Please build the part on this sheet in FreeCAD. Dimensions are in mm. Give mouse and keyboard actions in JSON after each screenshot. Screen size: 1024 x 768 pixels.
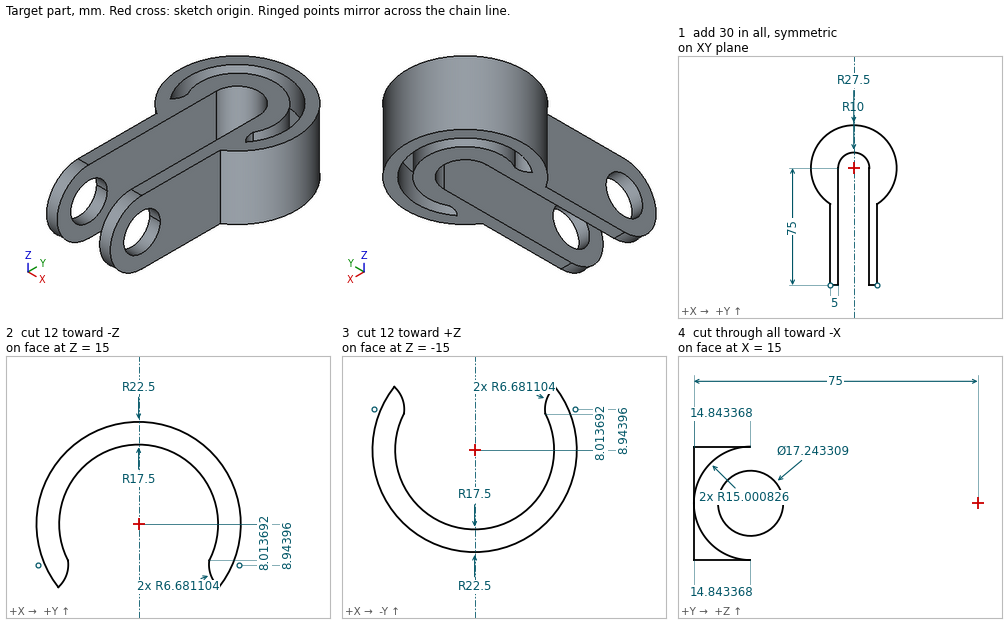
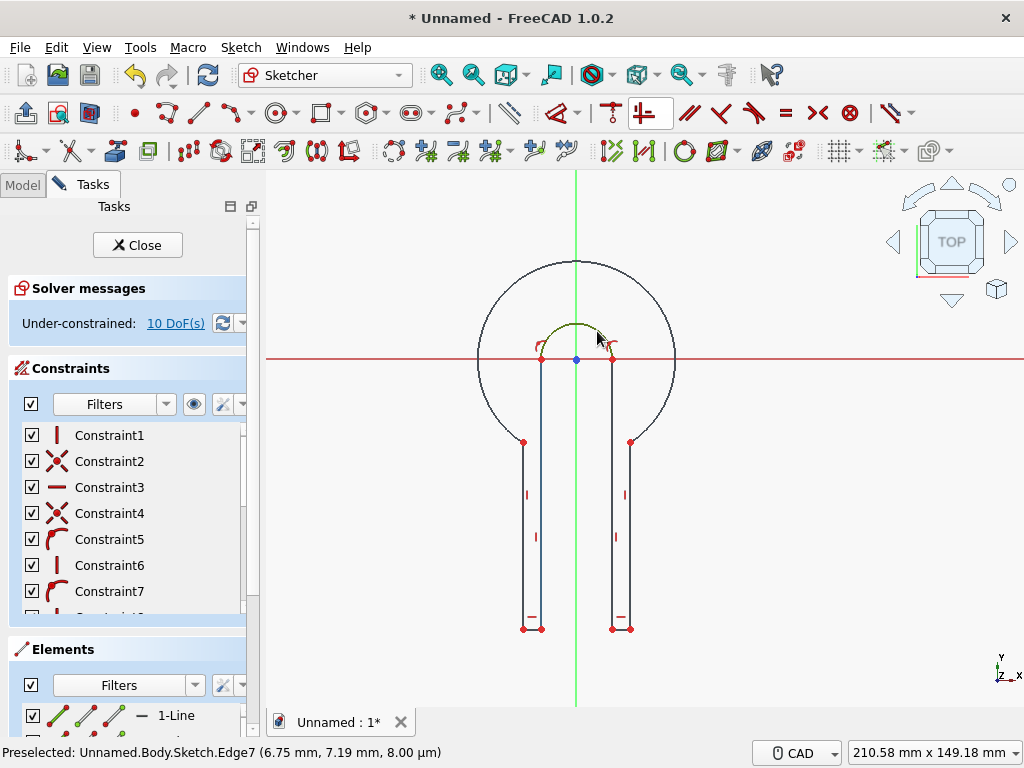
{"action": "key", "text": "t"}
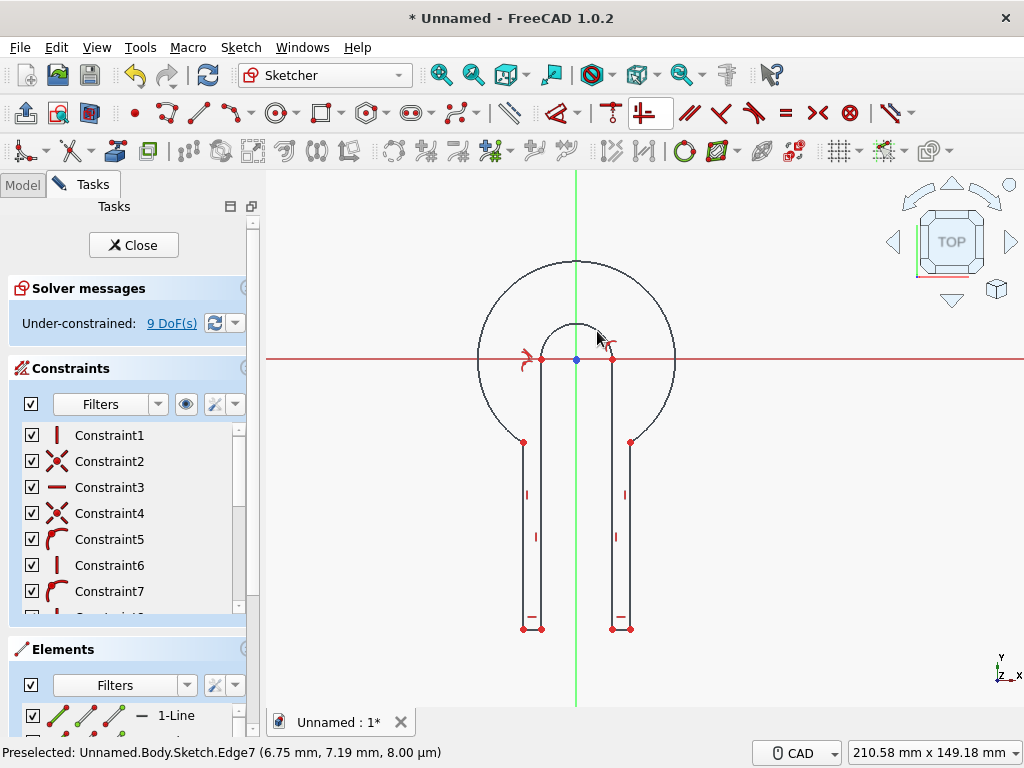
{"action": "left_click", "coordinate": [597, 331]}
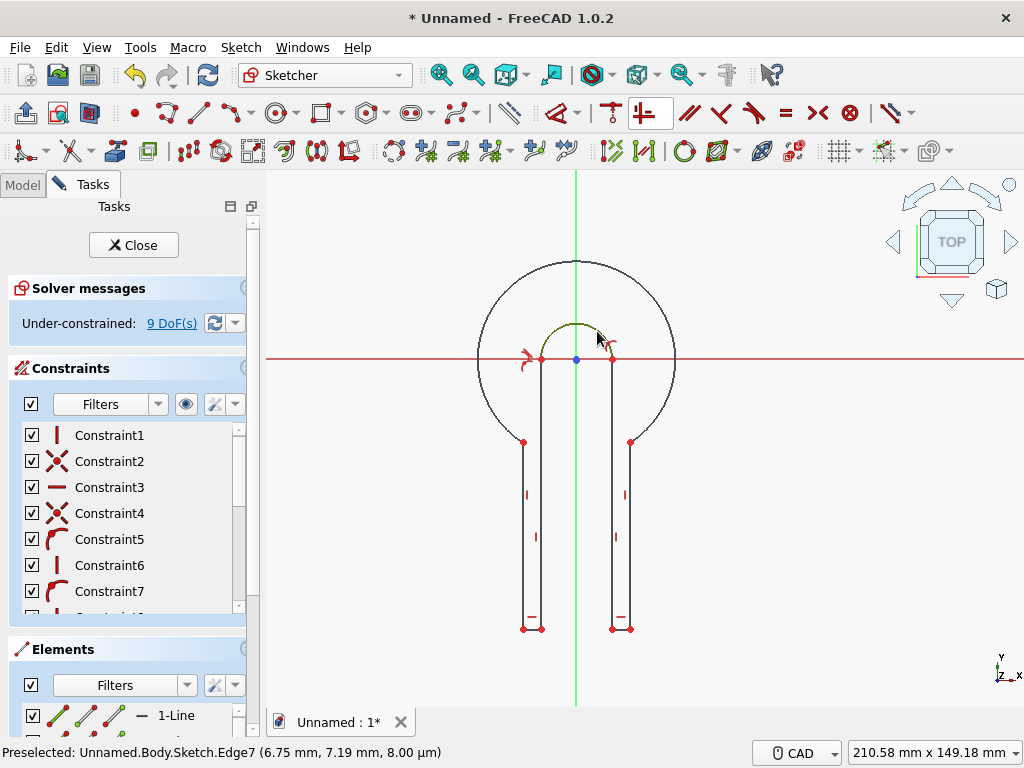
{"action": "left_click", "coordinate": [661, 309]}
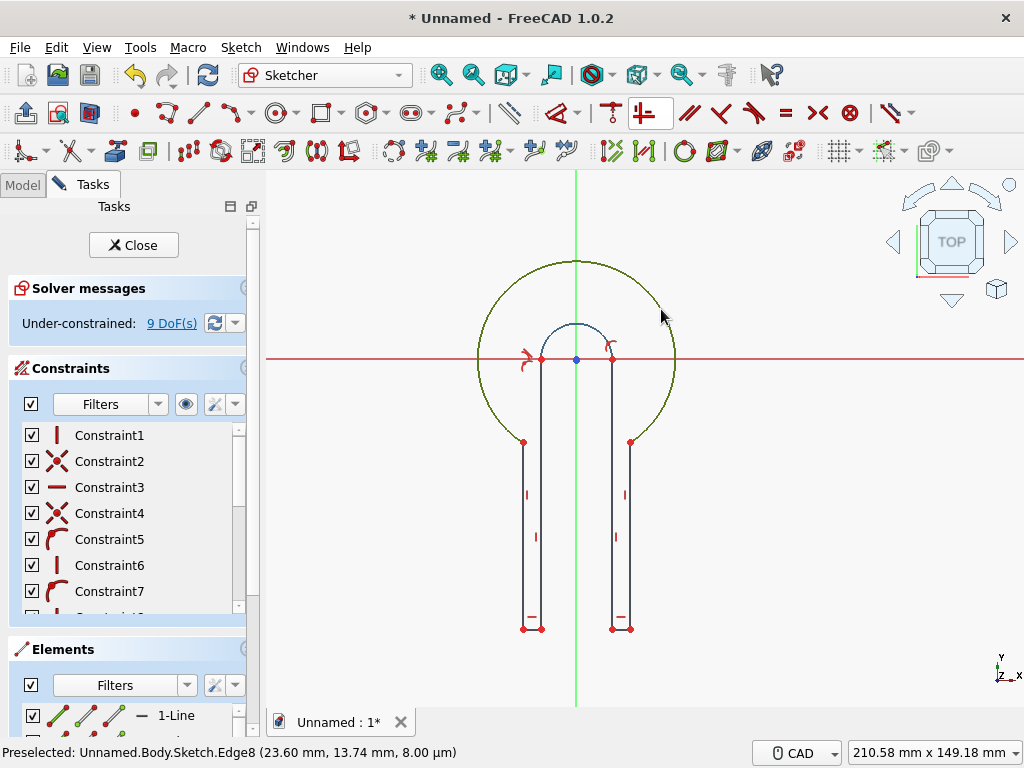
{"action": "key", "text": "c"}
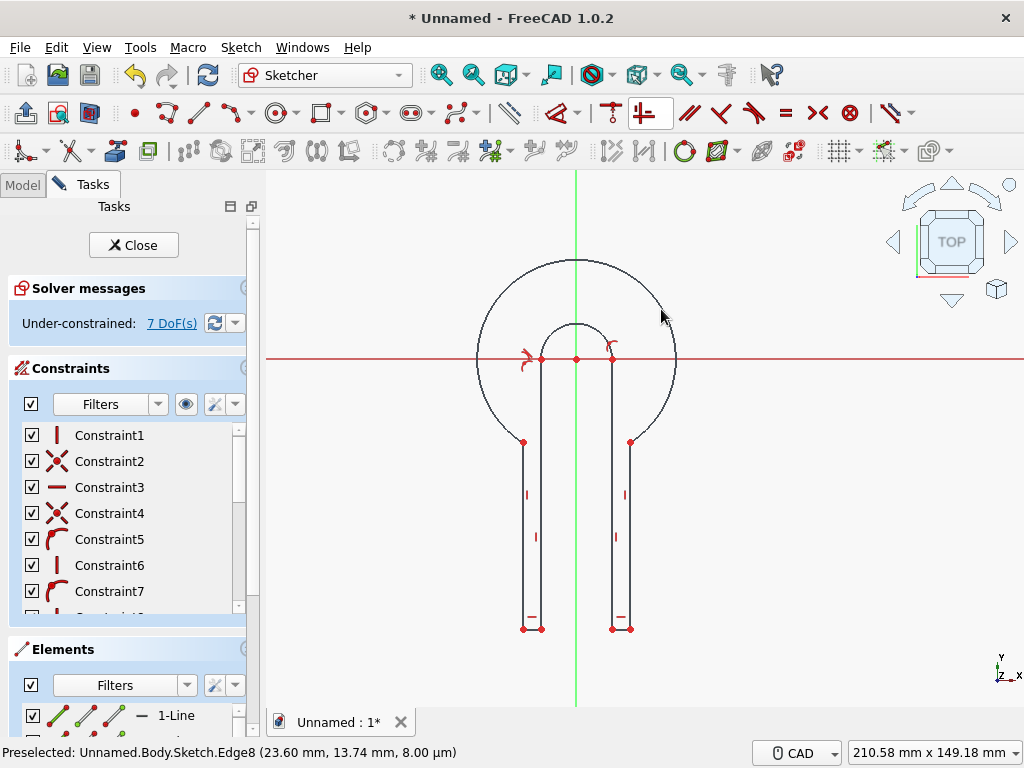
{"action": "left_click", "coordinate": [577, 359]}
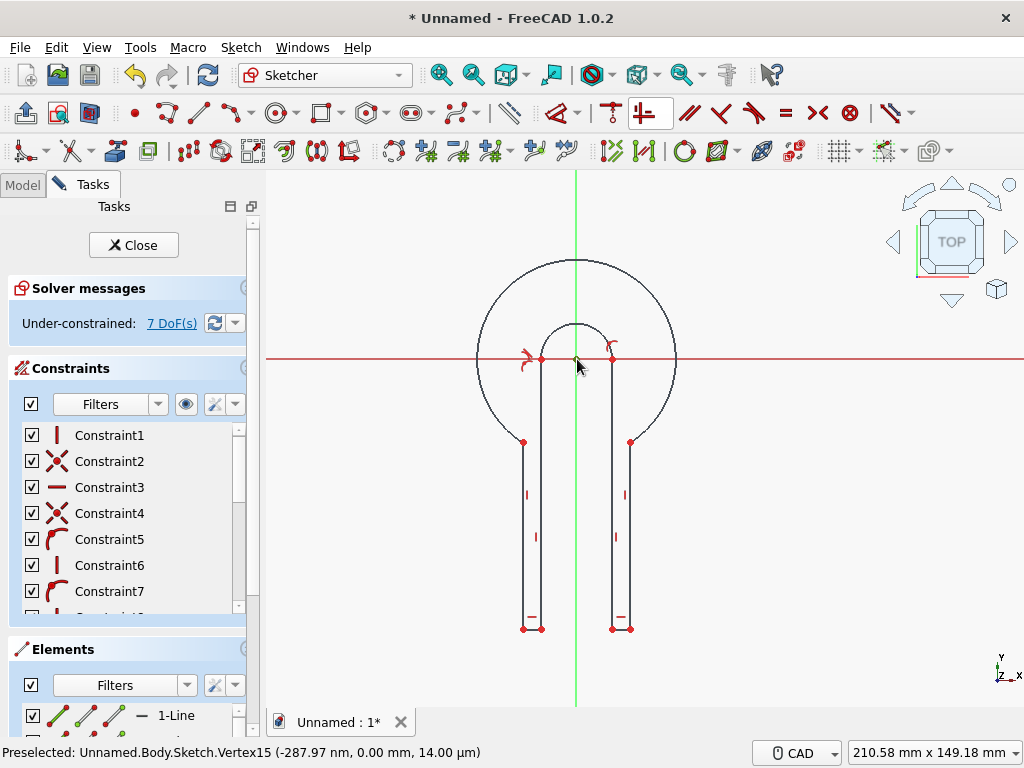
{"action": "left_click", "coordinate": [577, 645]}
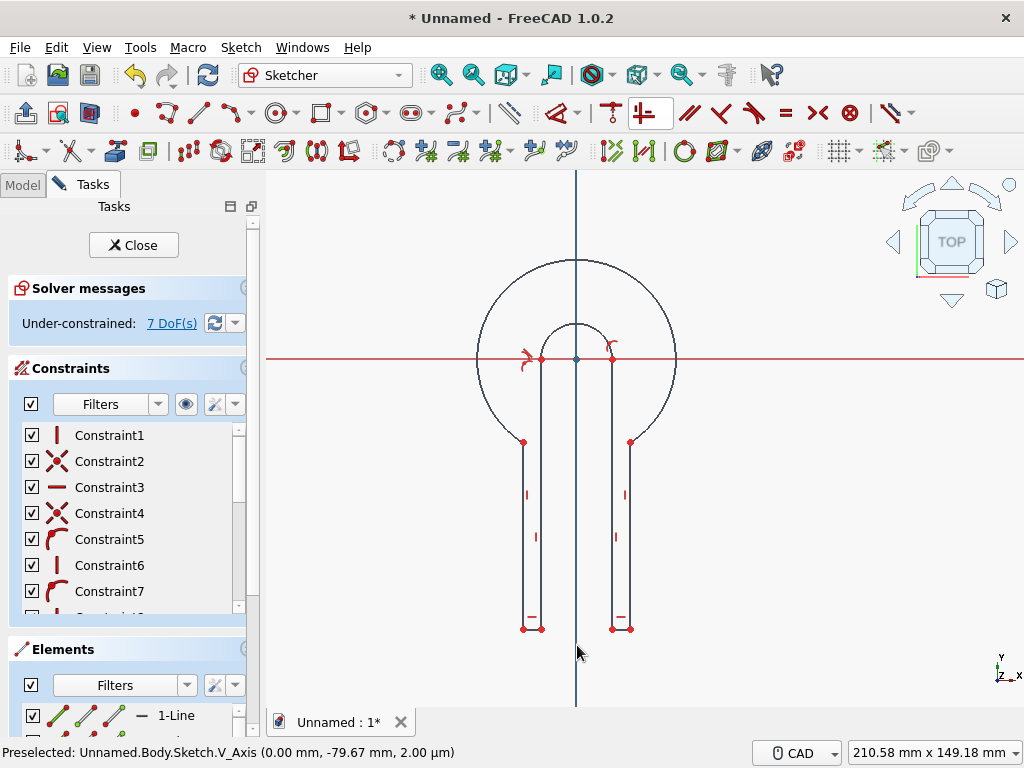
{"action": "key", "text": "c"}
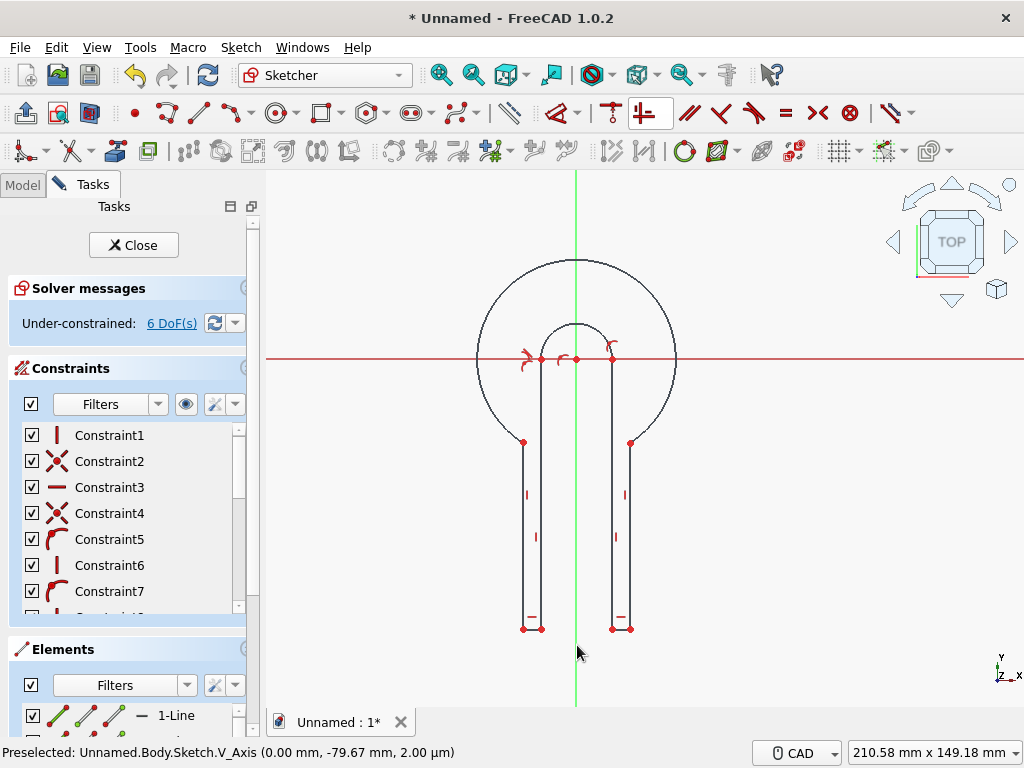
{"action": "left_click", "coordinate": [523, 630]}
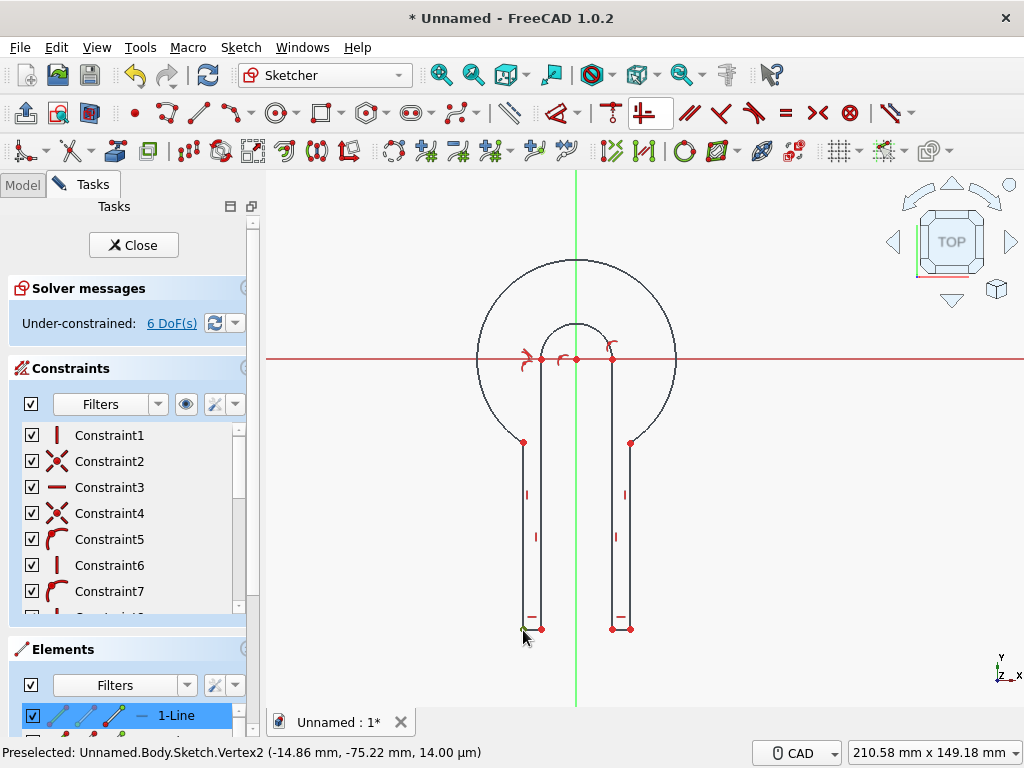
{"action": "left_click", "coordinate": [630, 630]}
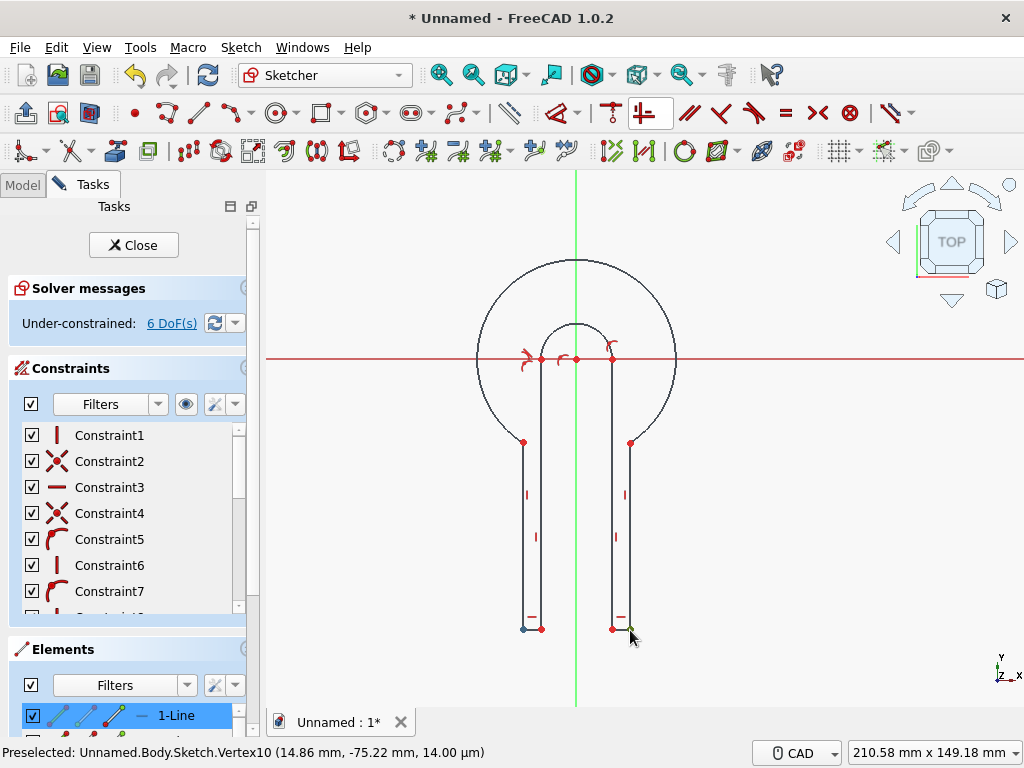
{"action": "left_click", "coordinate": [577, 645]}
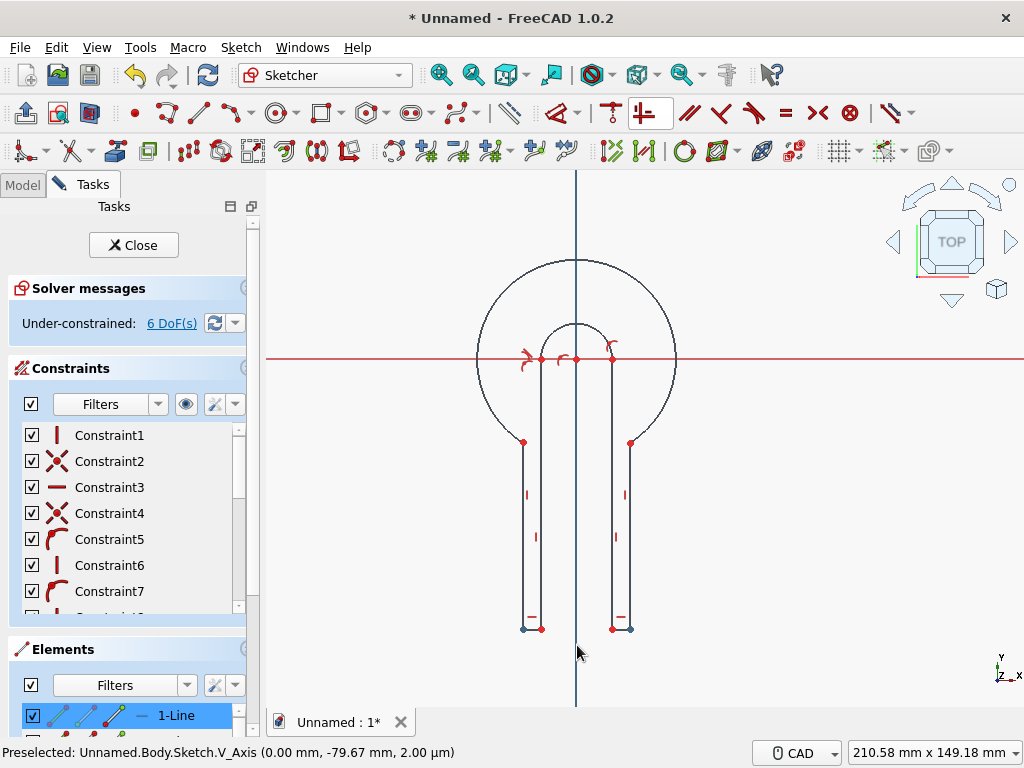
{"action": "key", "text": "s"}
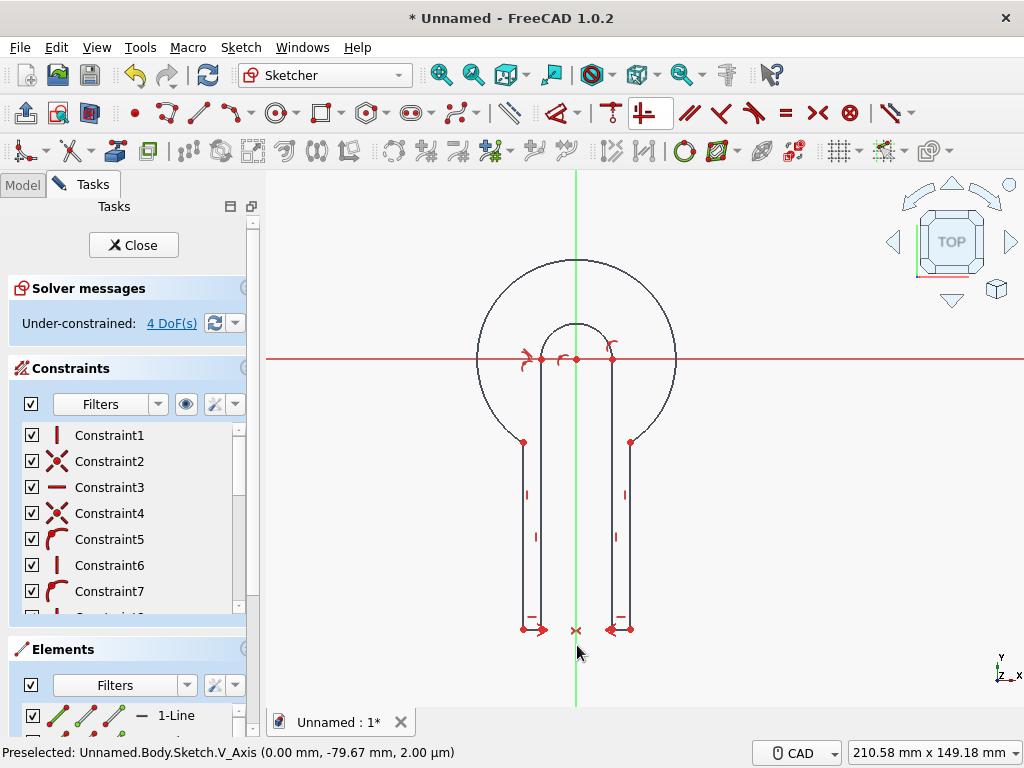
{"action": "left_click", "coordinate": [597, 331]}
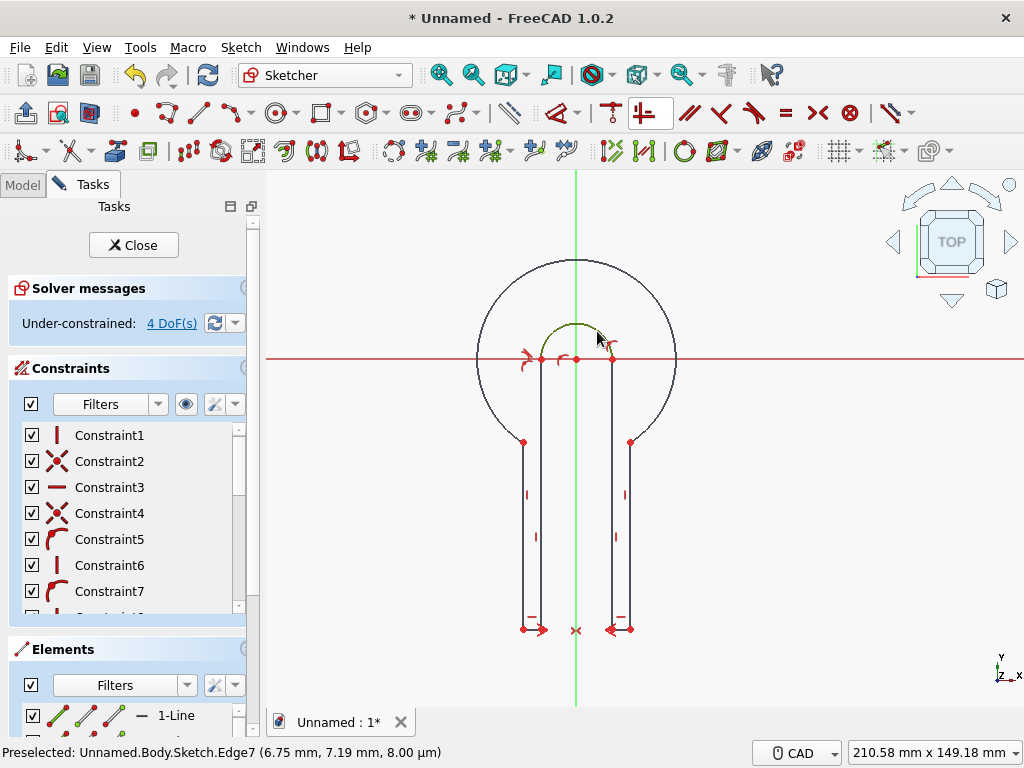
{"action": "key", "text": "k r"}